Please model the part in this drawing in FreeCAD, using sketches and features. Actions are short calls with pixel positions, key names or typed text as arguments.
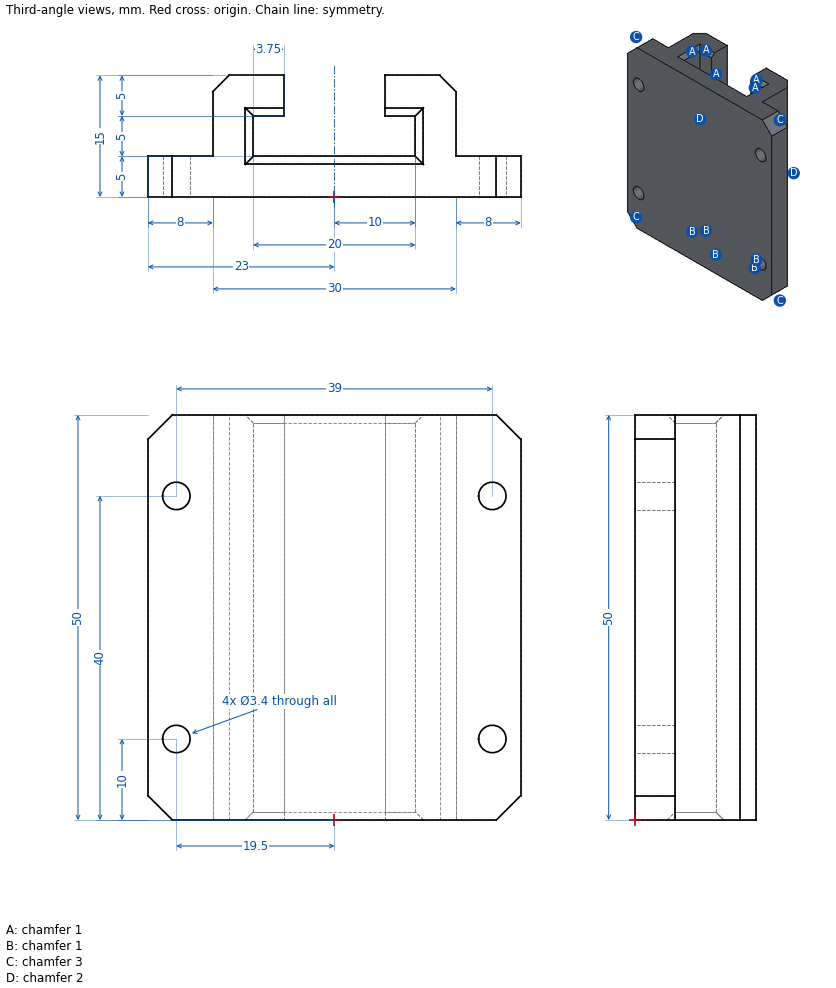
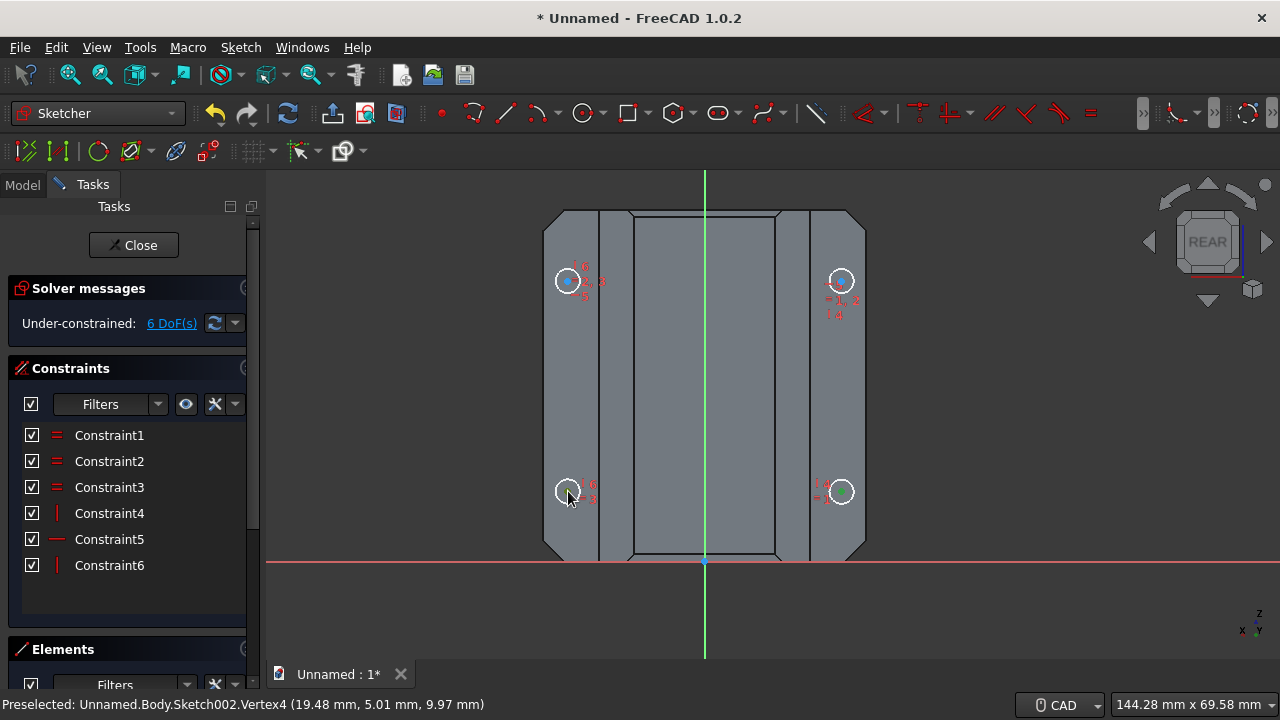
key(h)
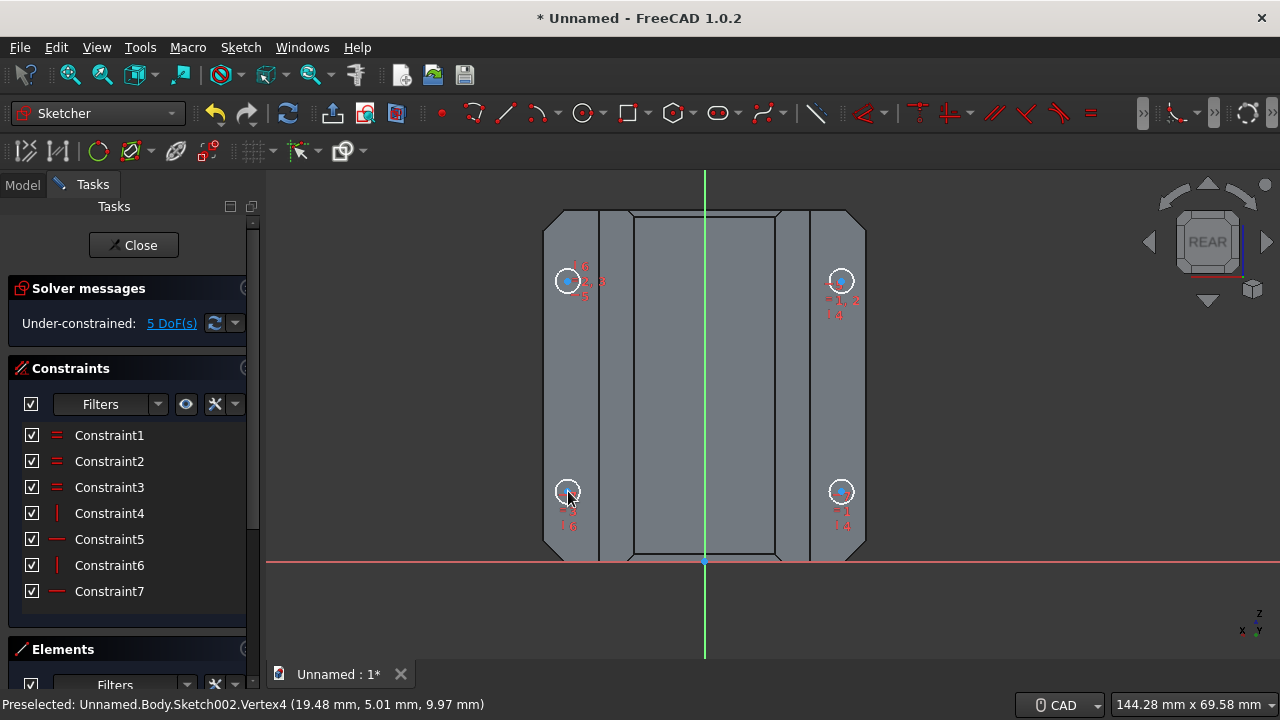
click(864, 114)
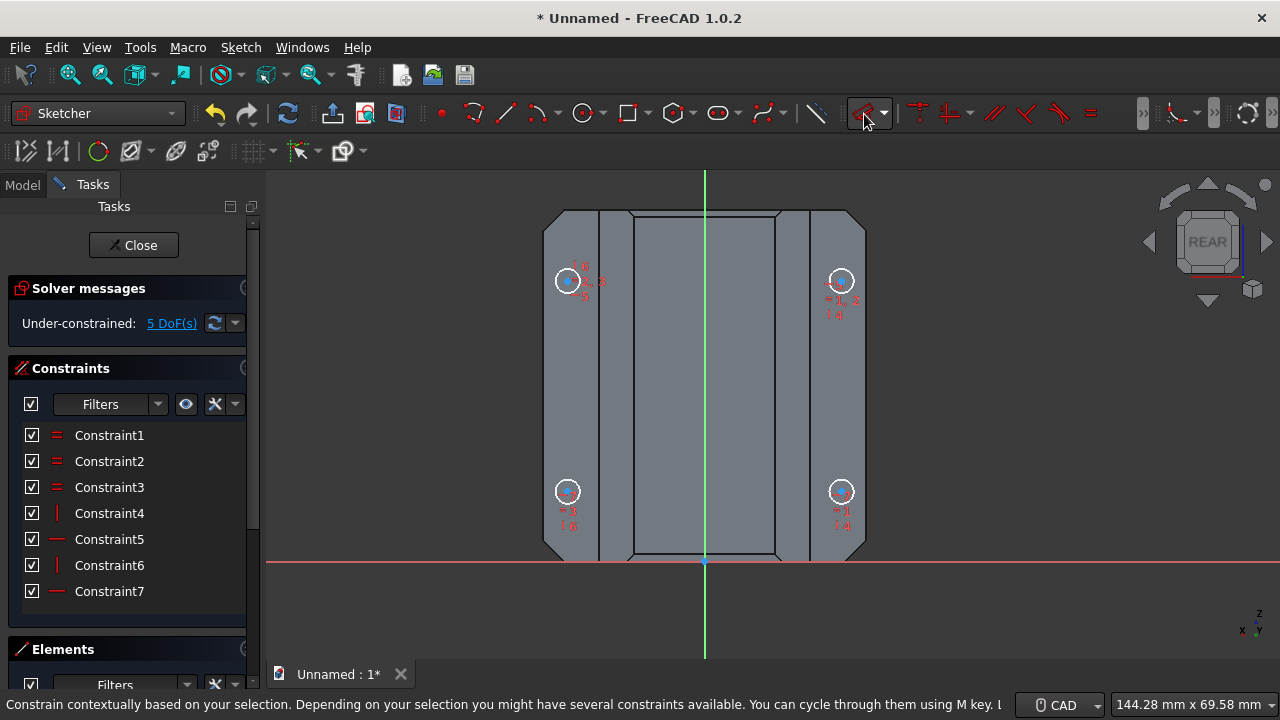
scroll(850, 483, up, 3)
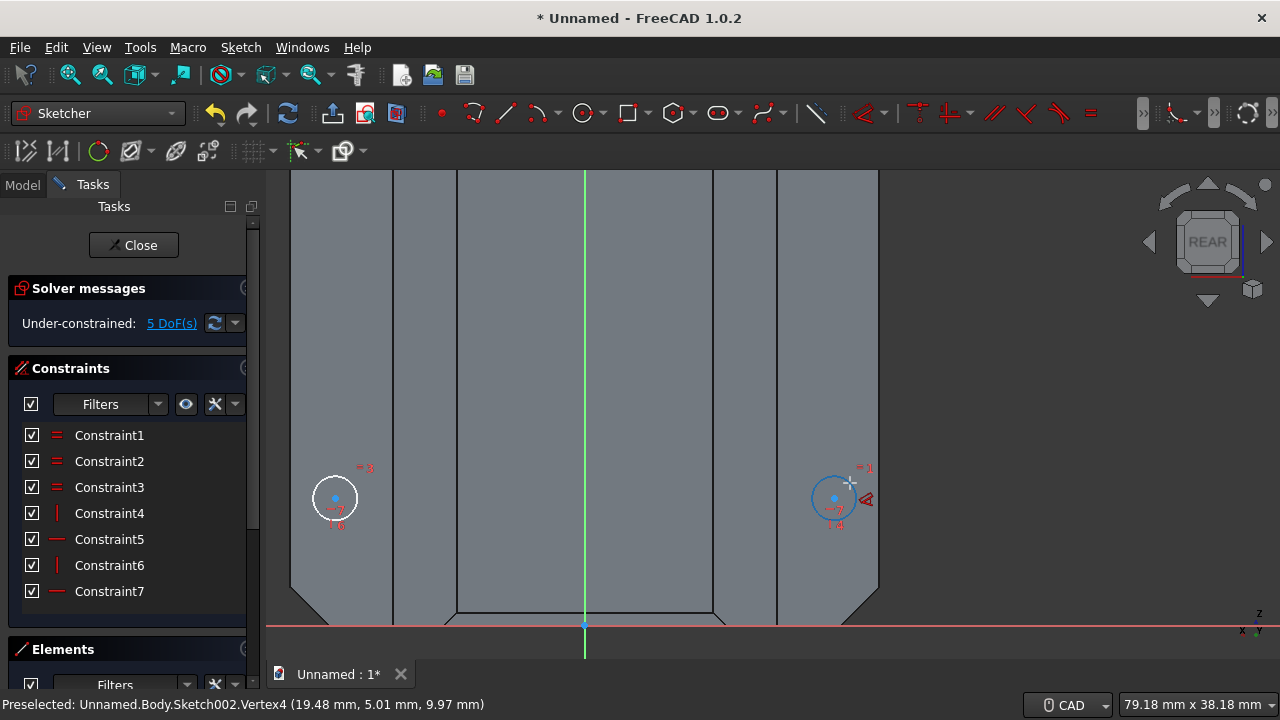
click(850, 483)
click(873, 461)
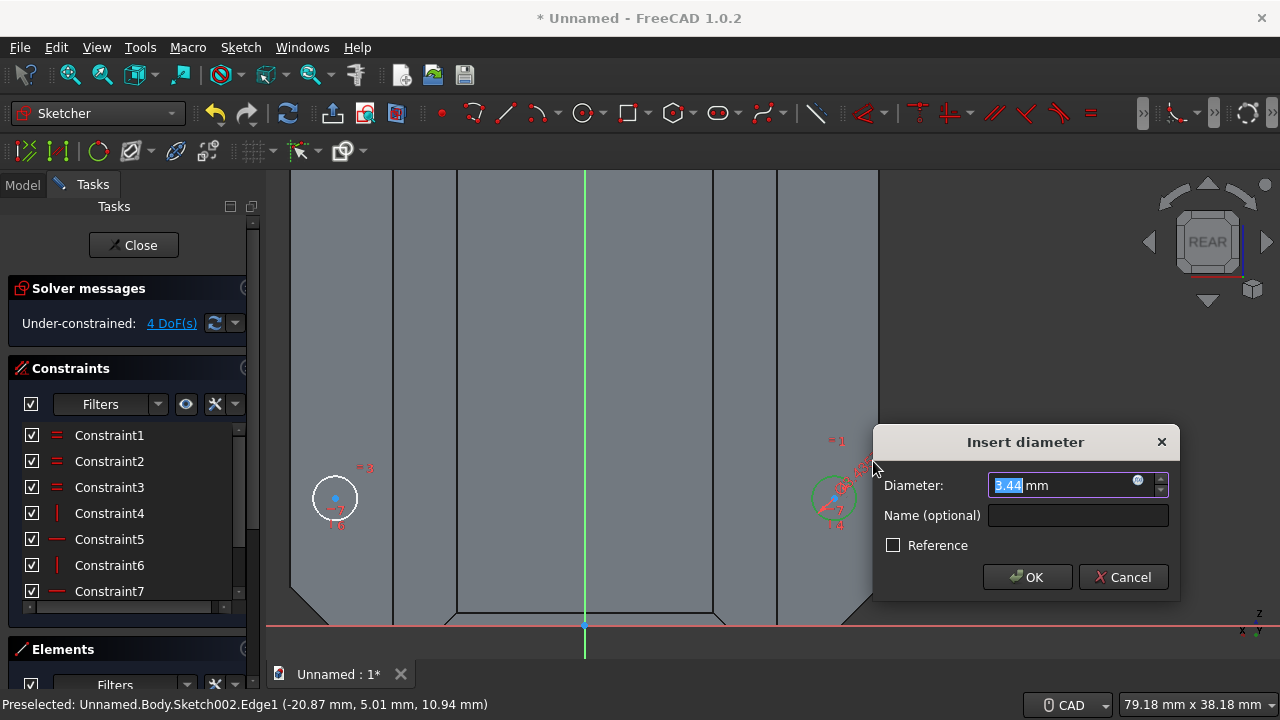
text(3.4)
key(Return)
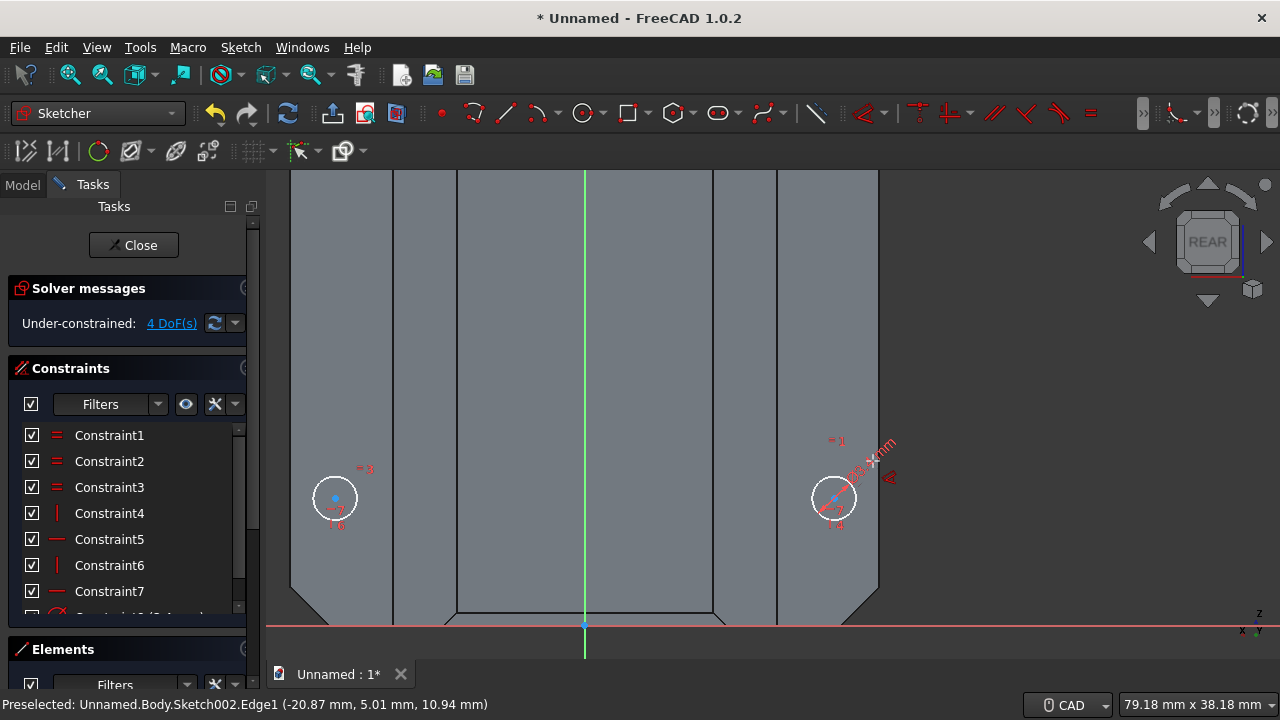
click(834, 498)
click(868, 562)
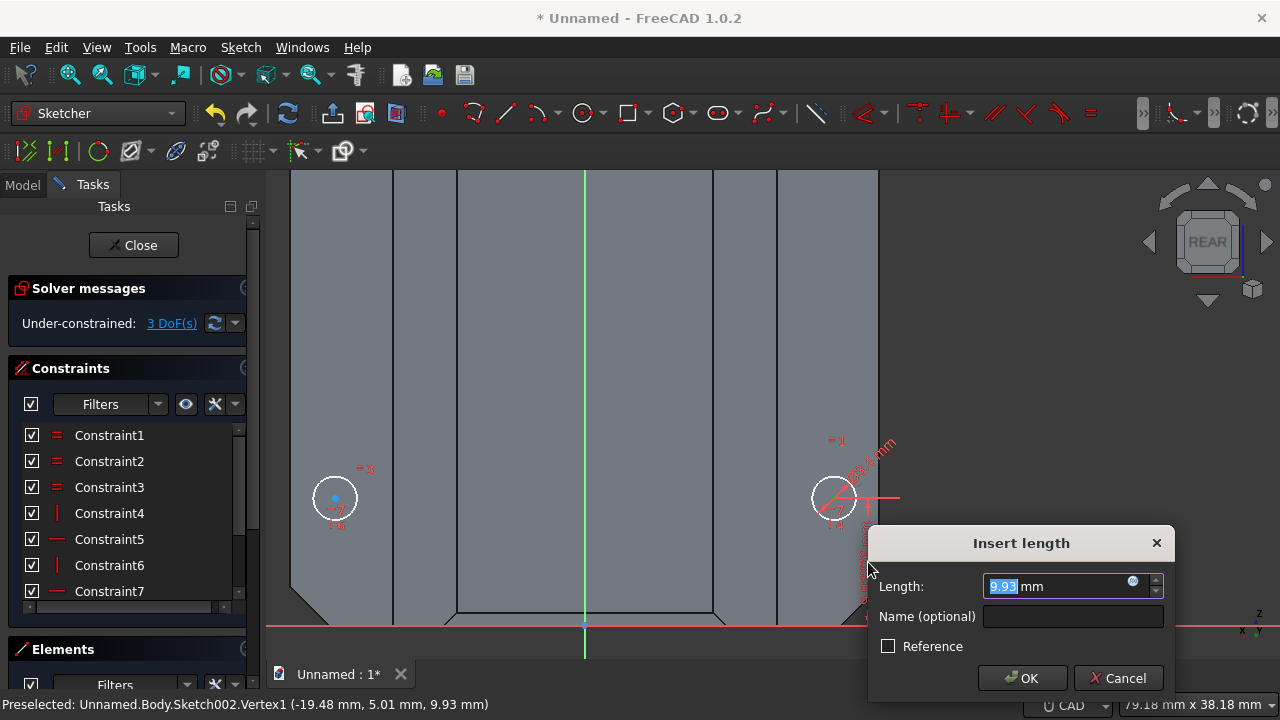
text(10)
key(Return)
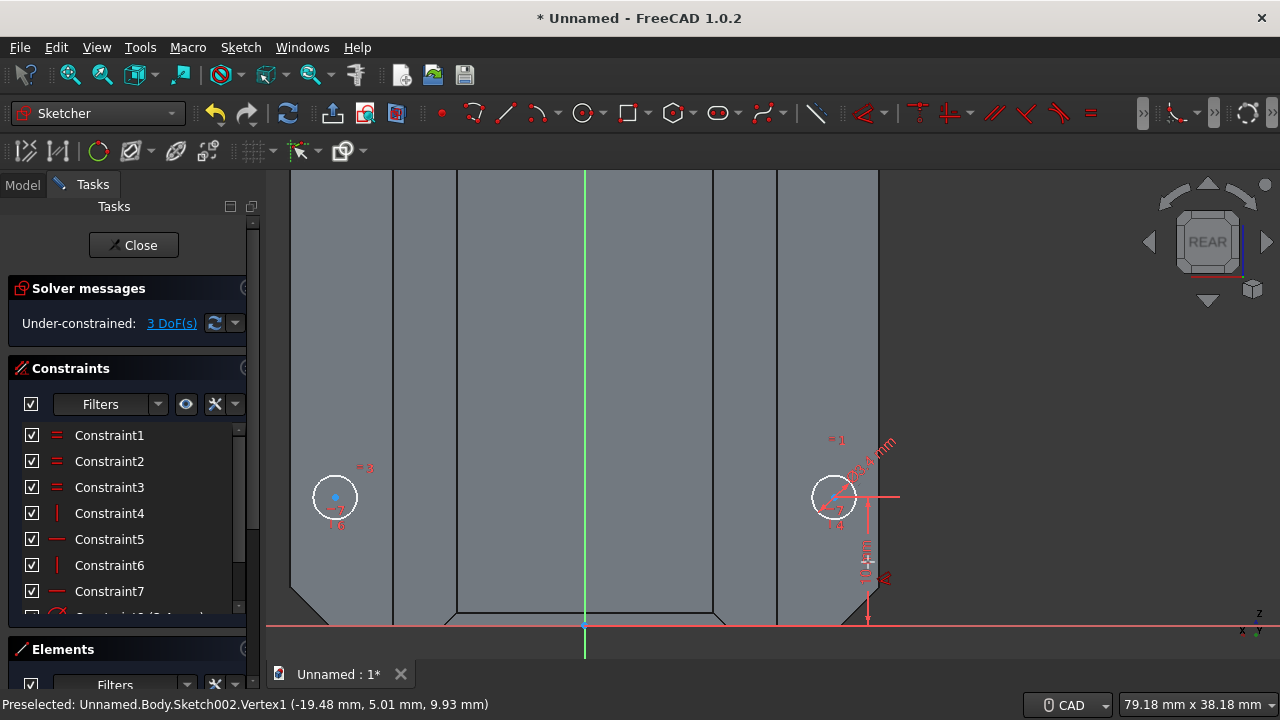
scroll(850, 483, down, 3)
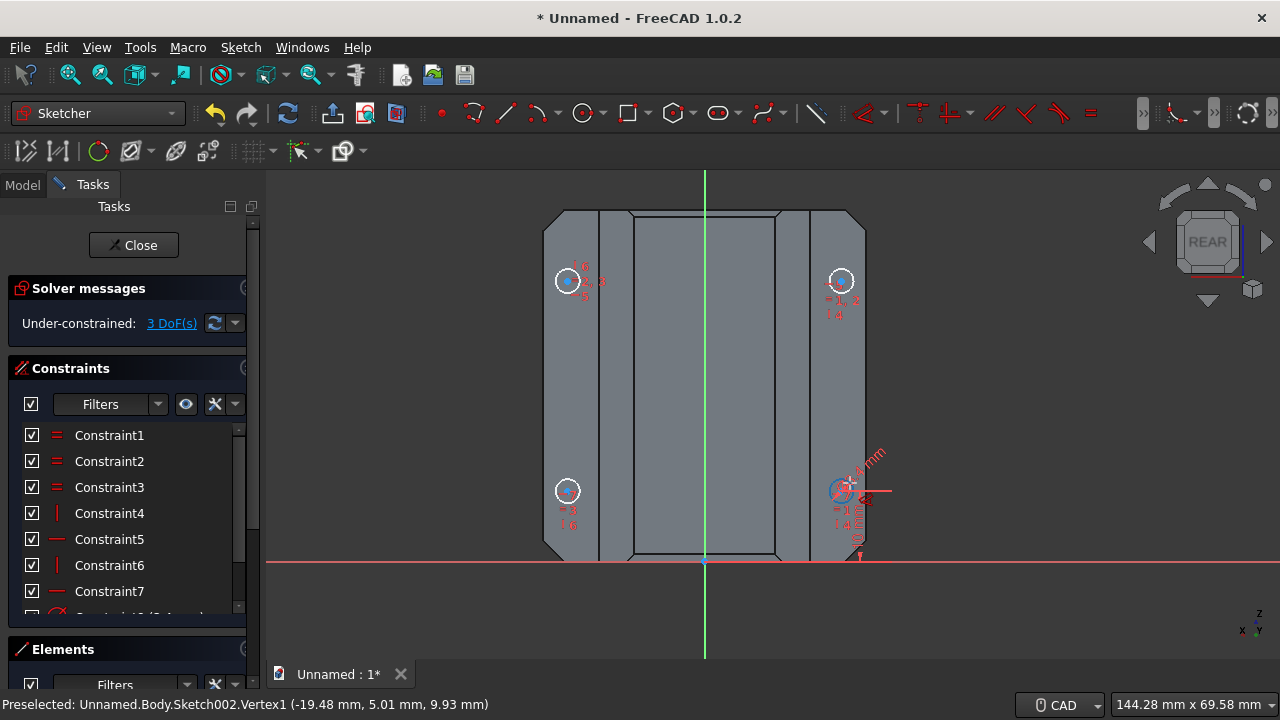
click(842, 281)
click(876, 421)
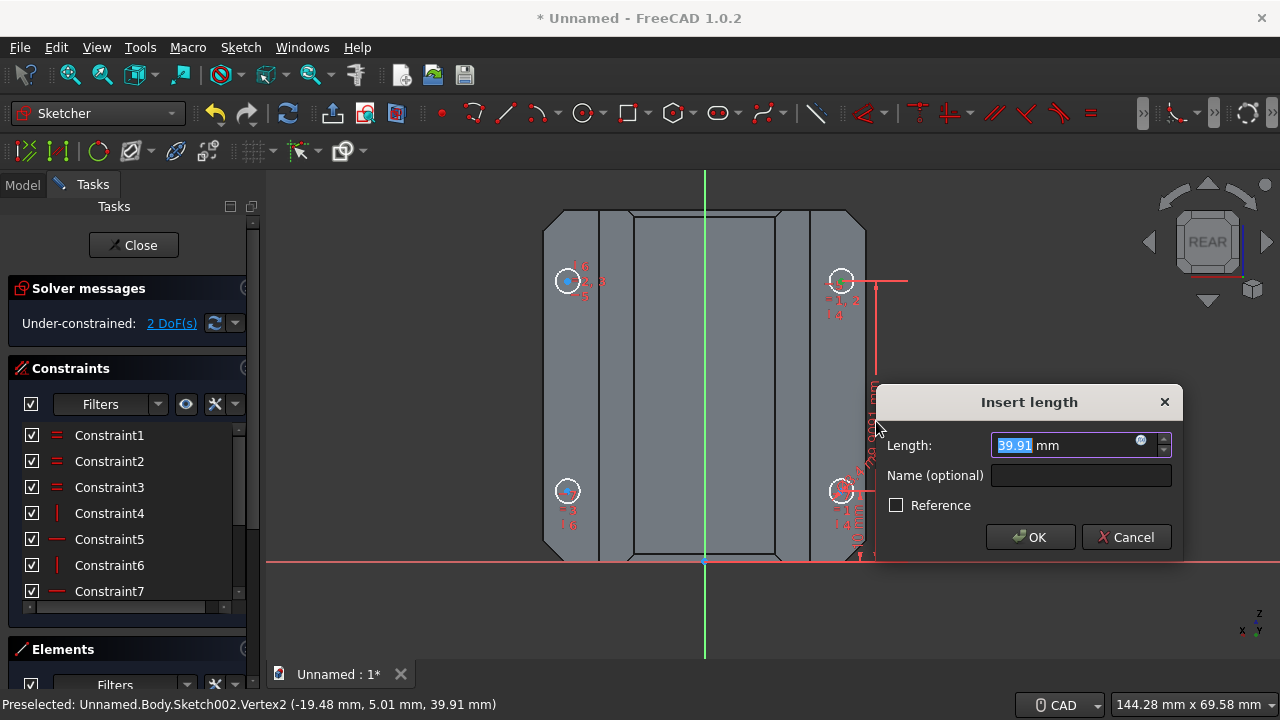
text(40)
key(Return)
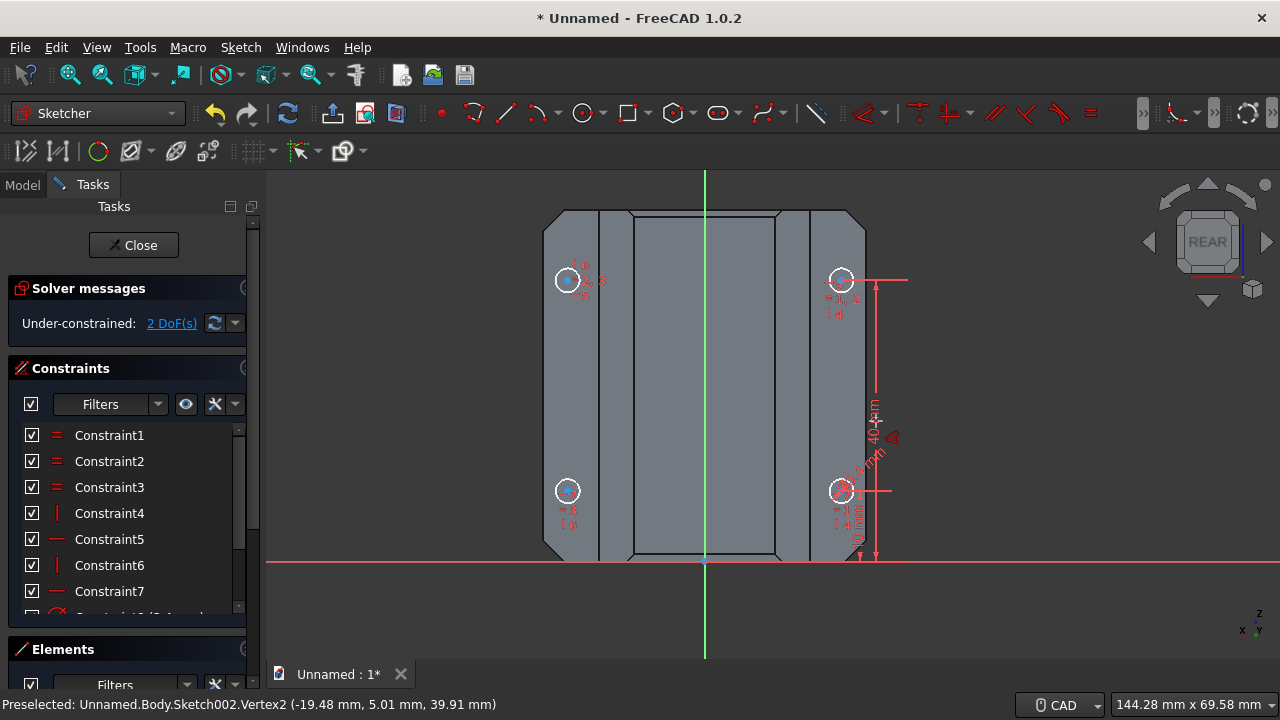
click(842, 280)